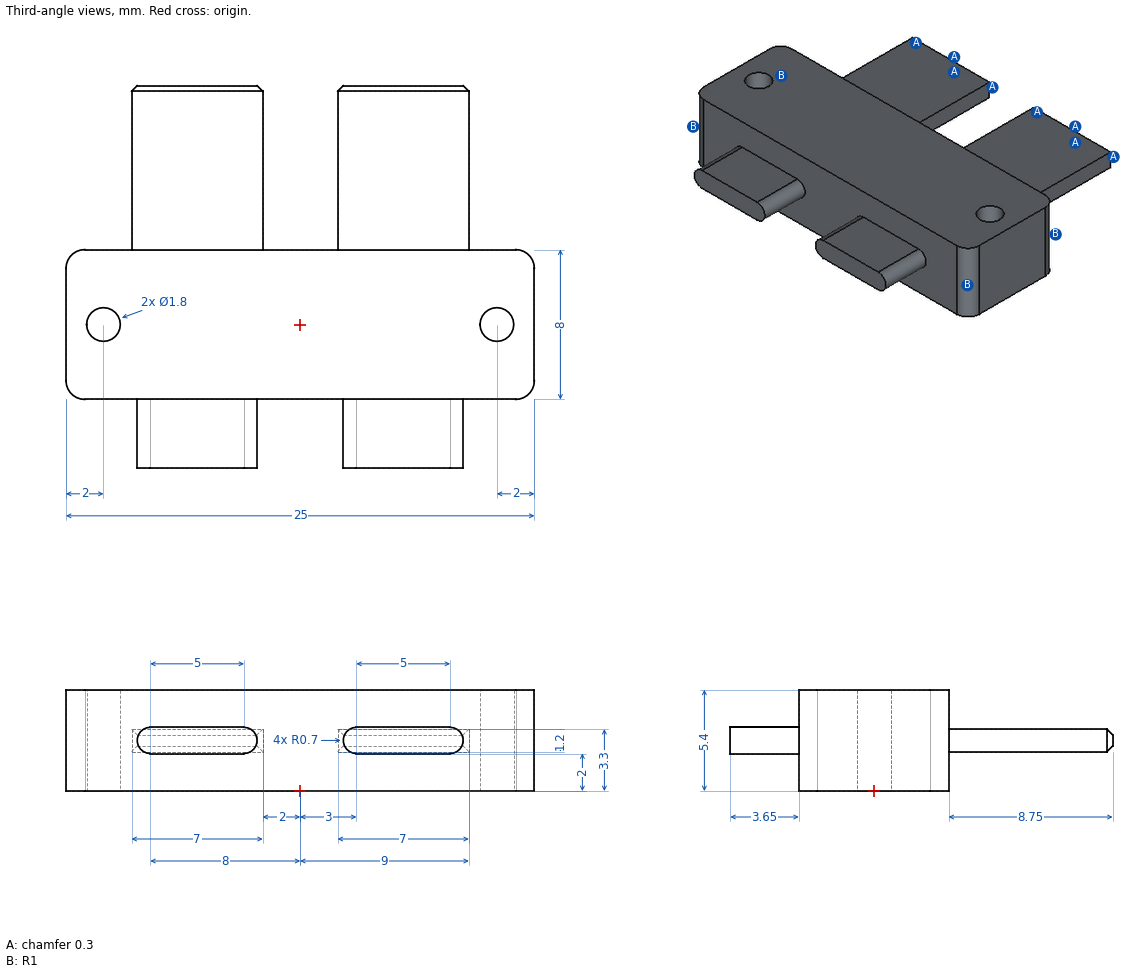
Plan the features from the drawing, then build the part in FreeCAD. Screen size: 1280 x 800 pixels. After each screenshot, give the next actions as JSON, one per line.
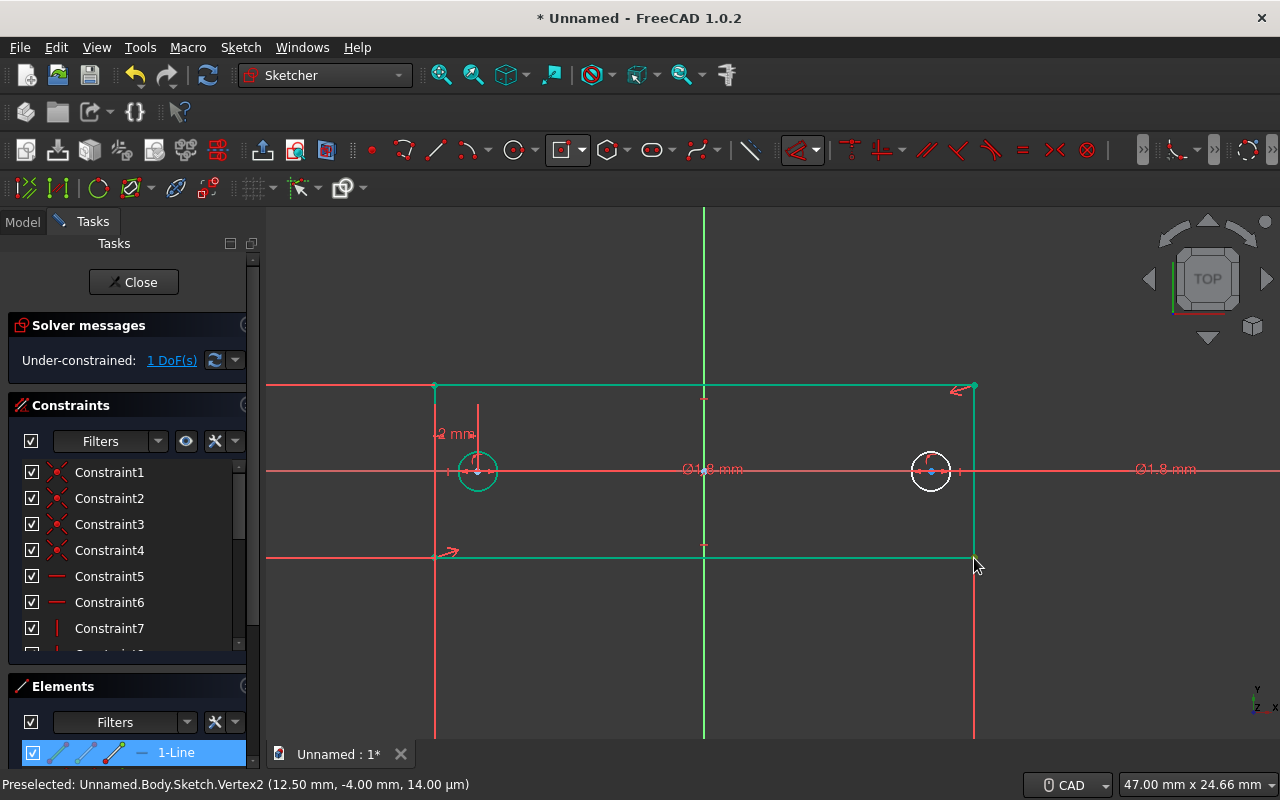
{"action": "left_click", "coordinate": [931, 471]}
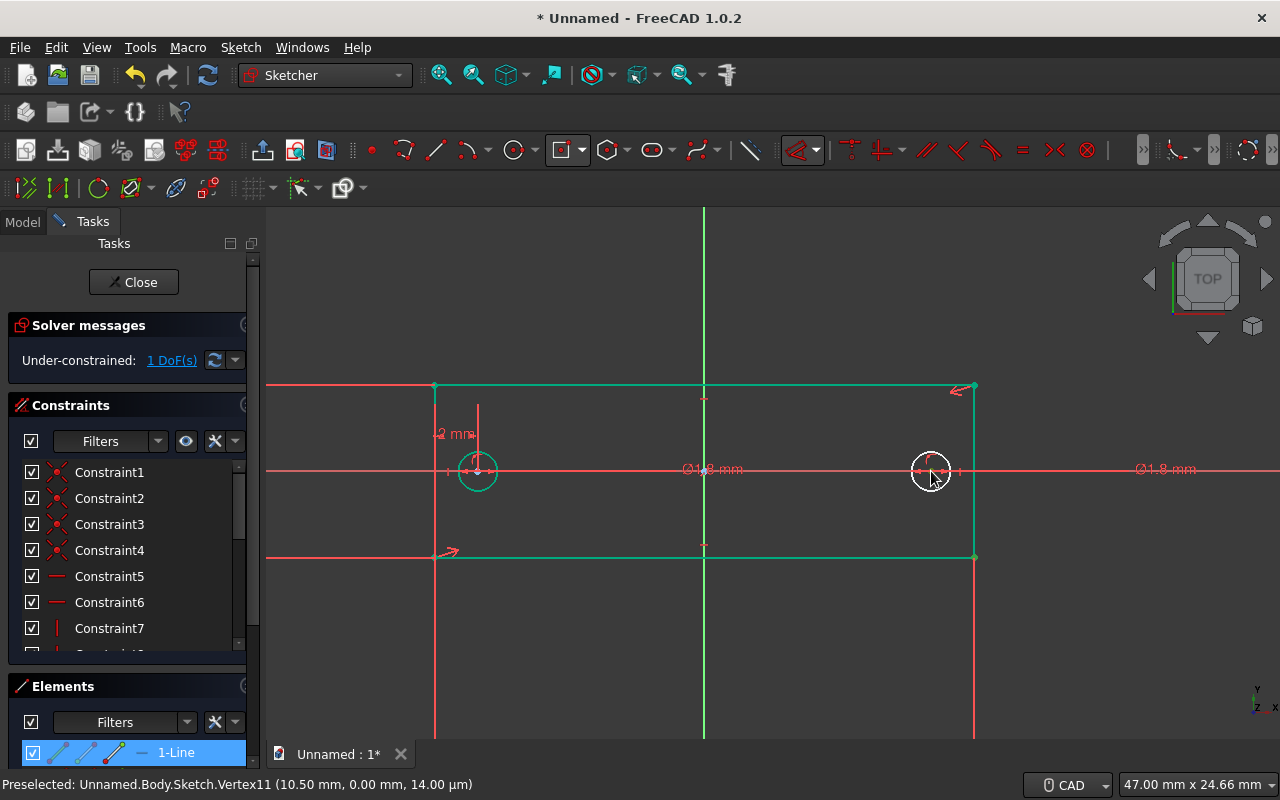
{"action": "key", "text": "l"}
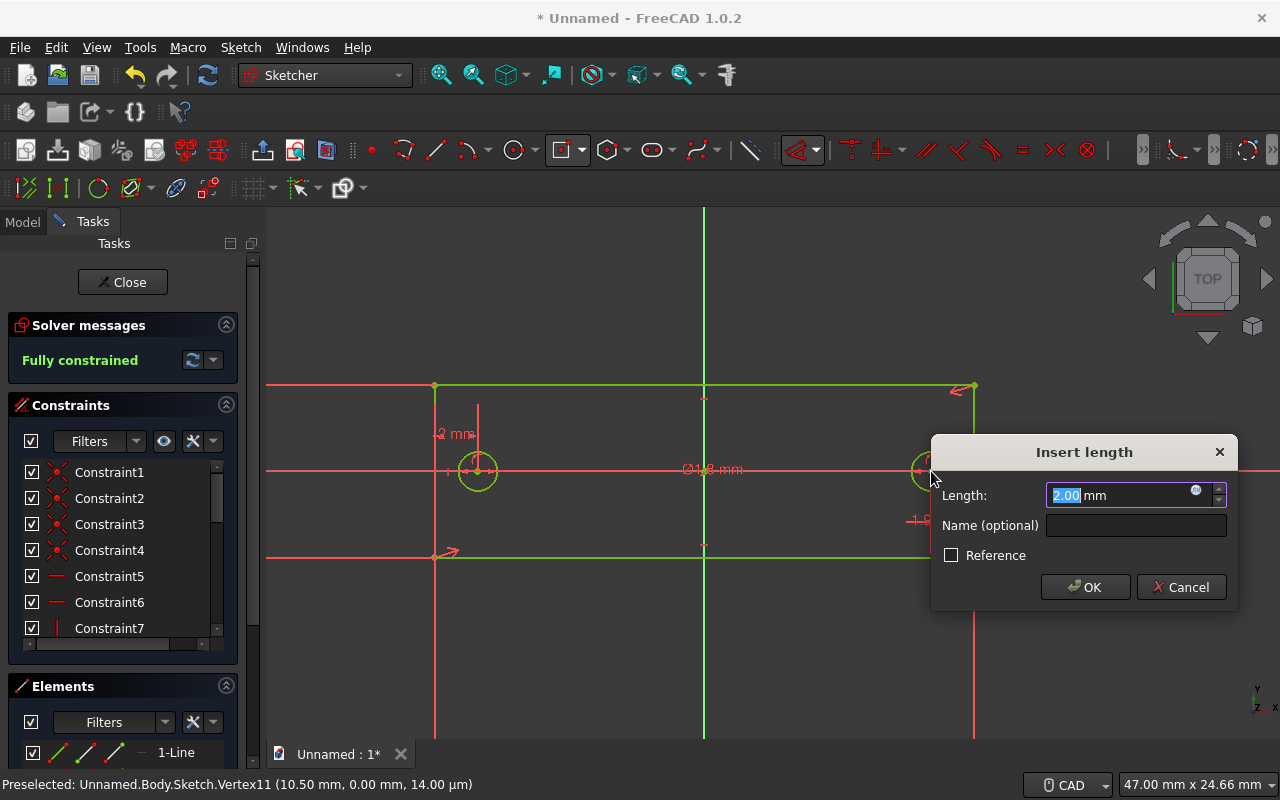
{"action": "type", "text": "2"}
{"action": "key", "text": "Return"}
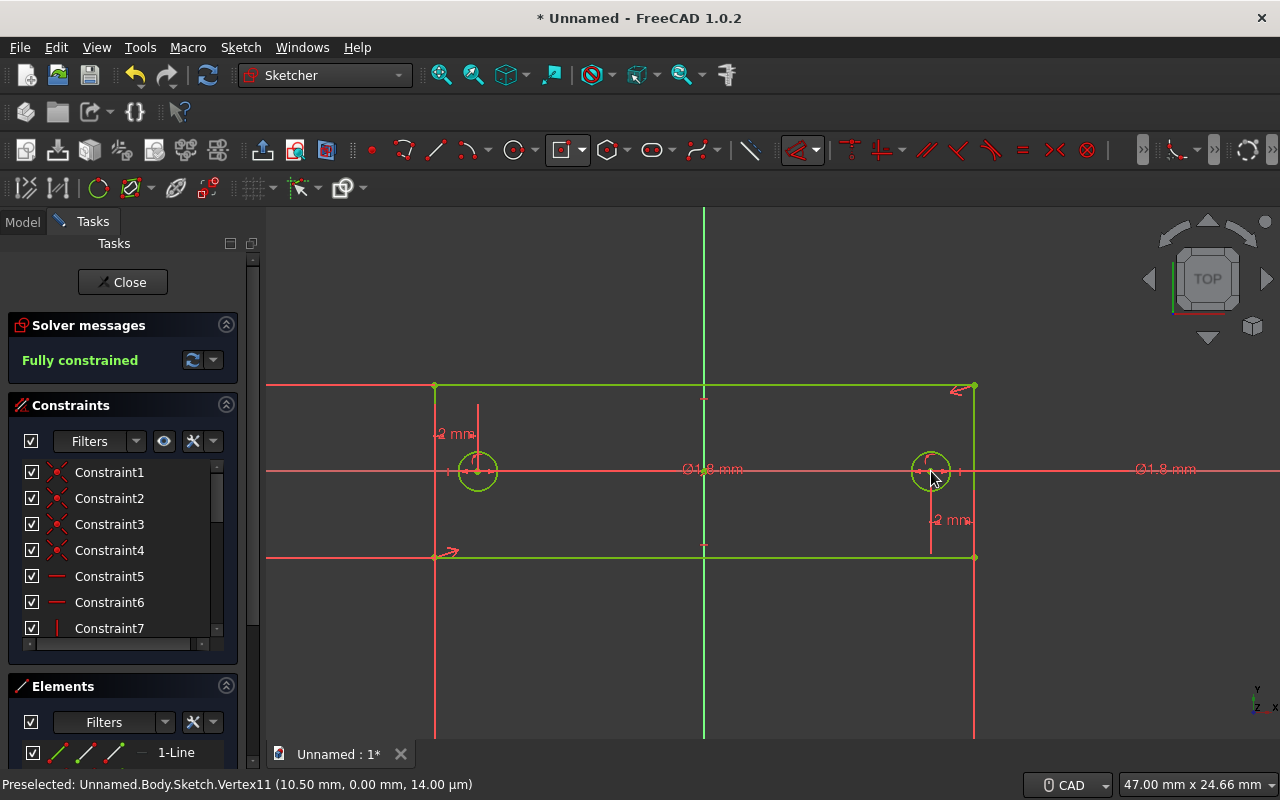
{"action": "left_click", "coordinate": [123, 282]}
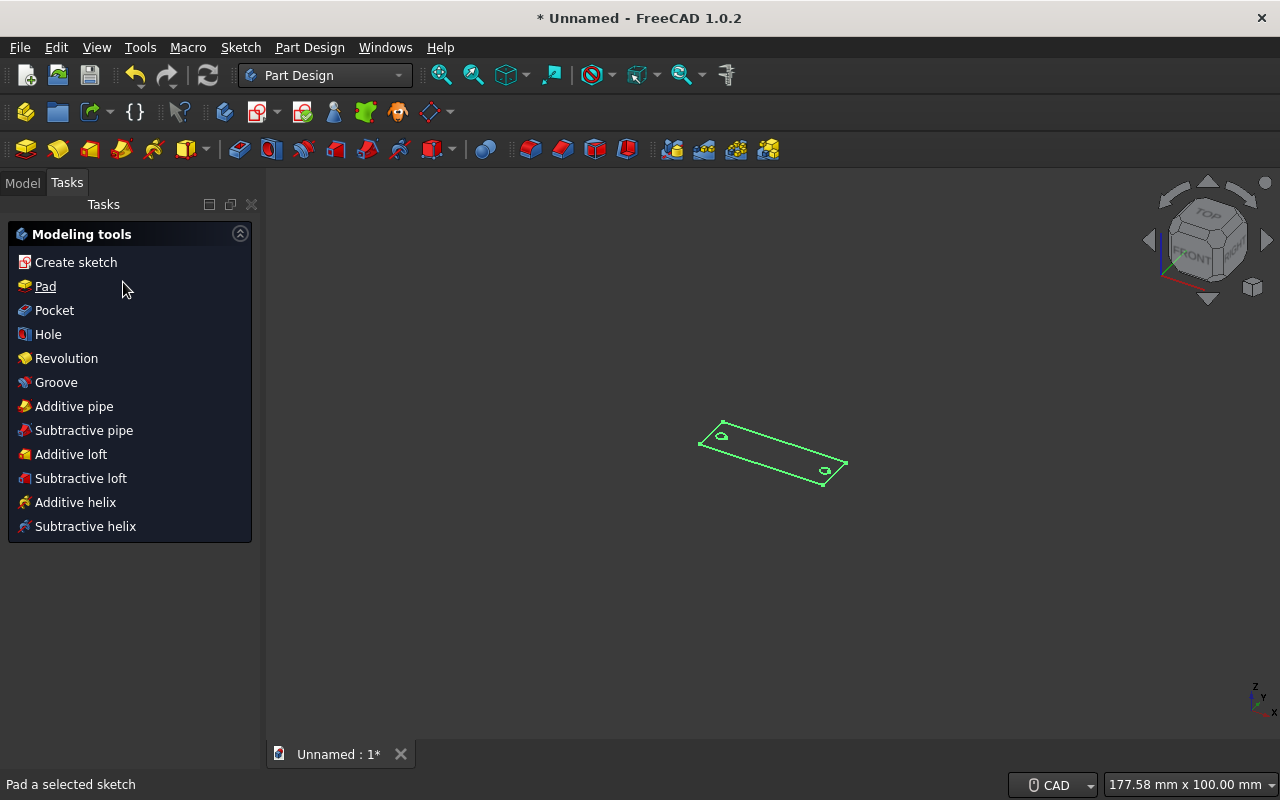
{"action": "left_click", "coordinate": [26, 150]}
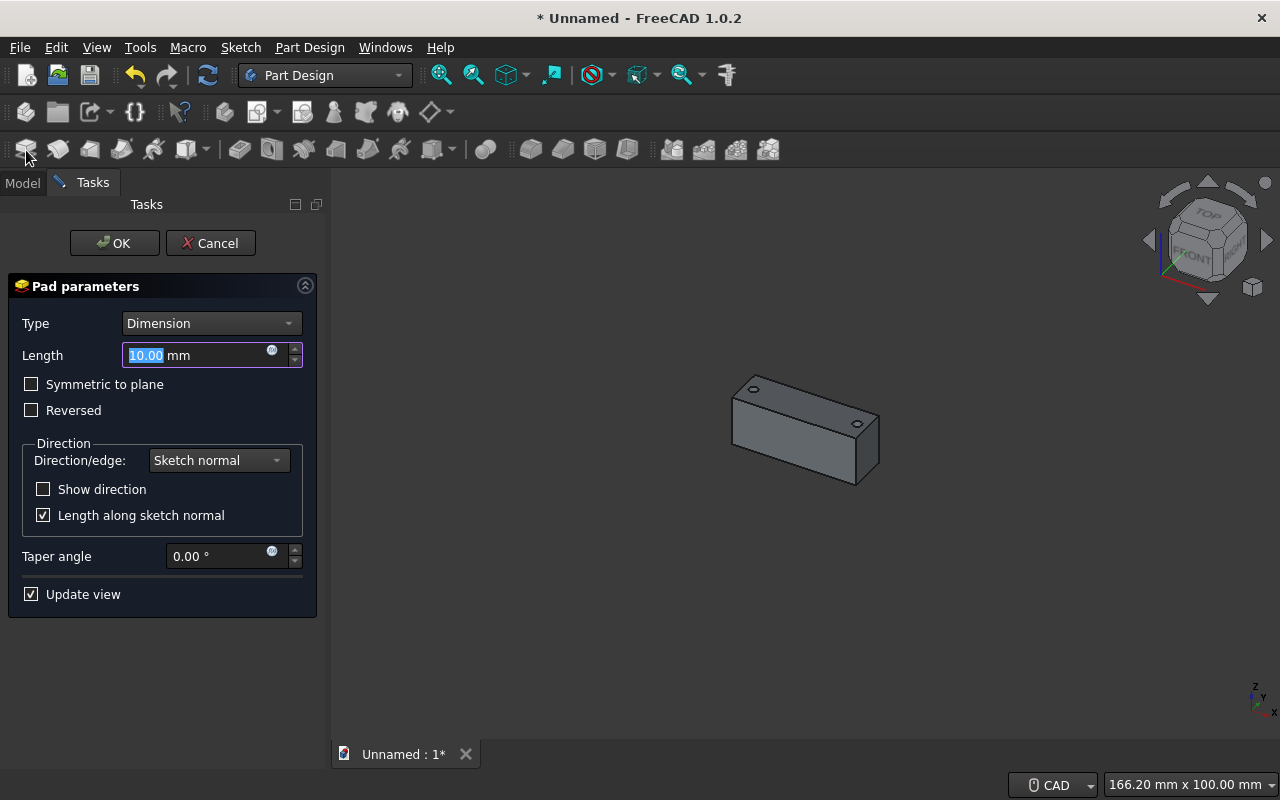
{"action": "type", "text": "5.4"}
{"action": "key", "text": "Tab"}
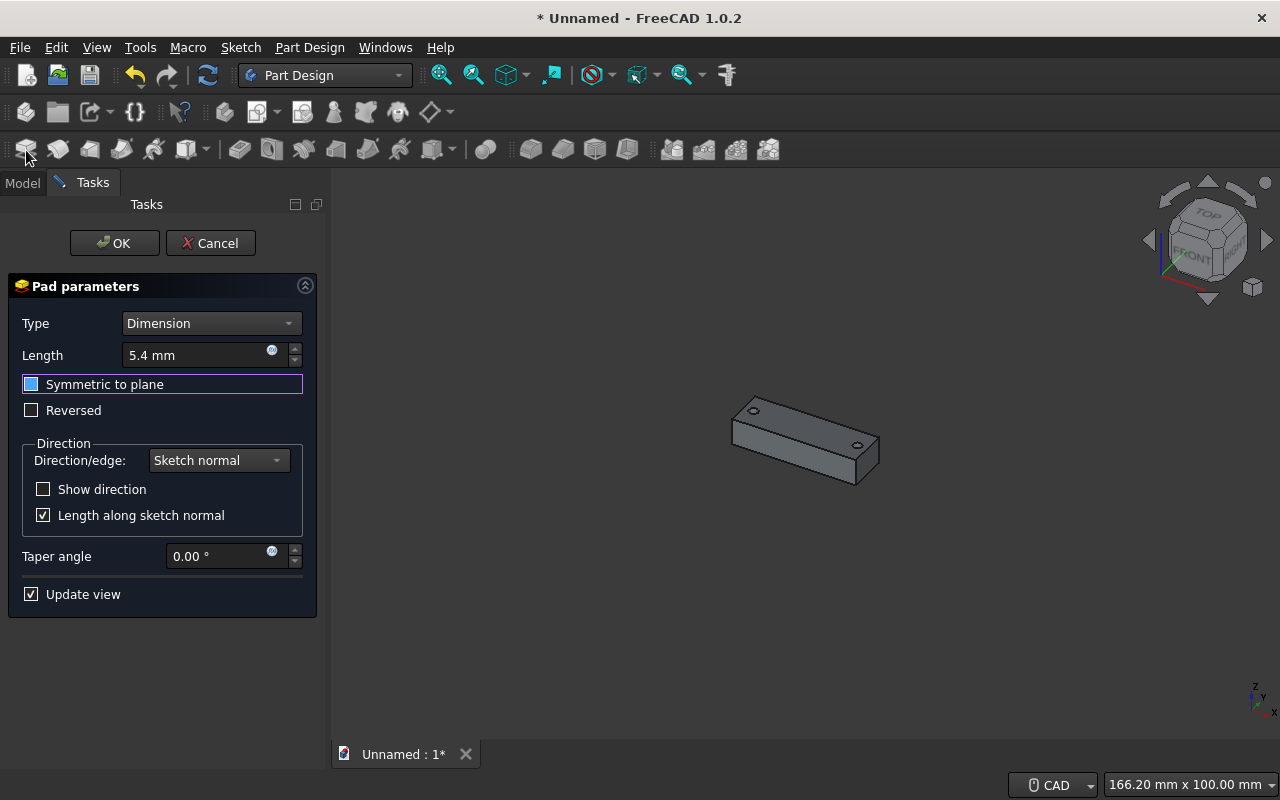
{"action": "left_click", "coordinate": [115, 243]}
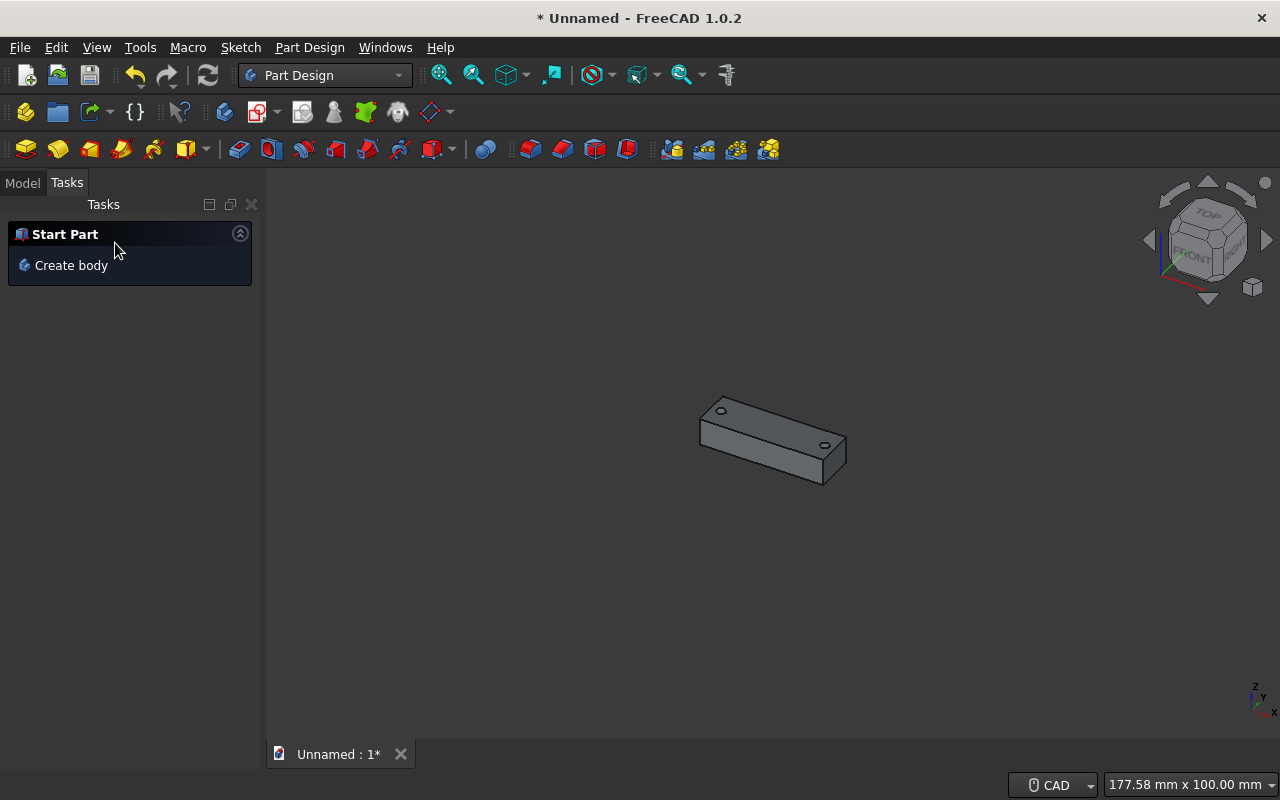
{"action": "left_click", "coordinate": [442, 76]}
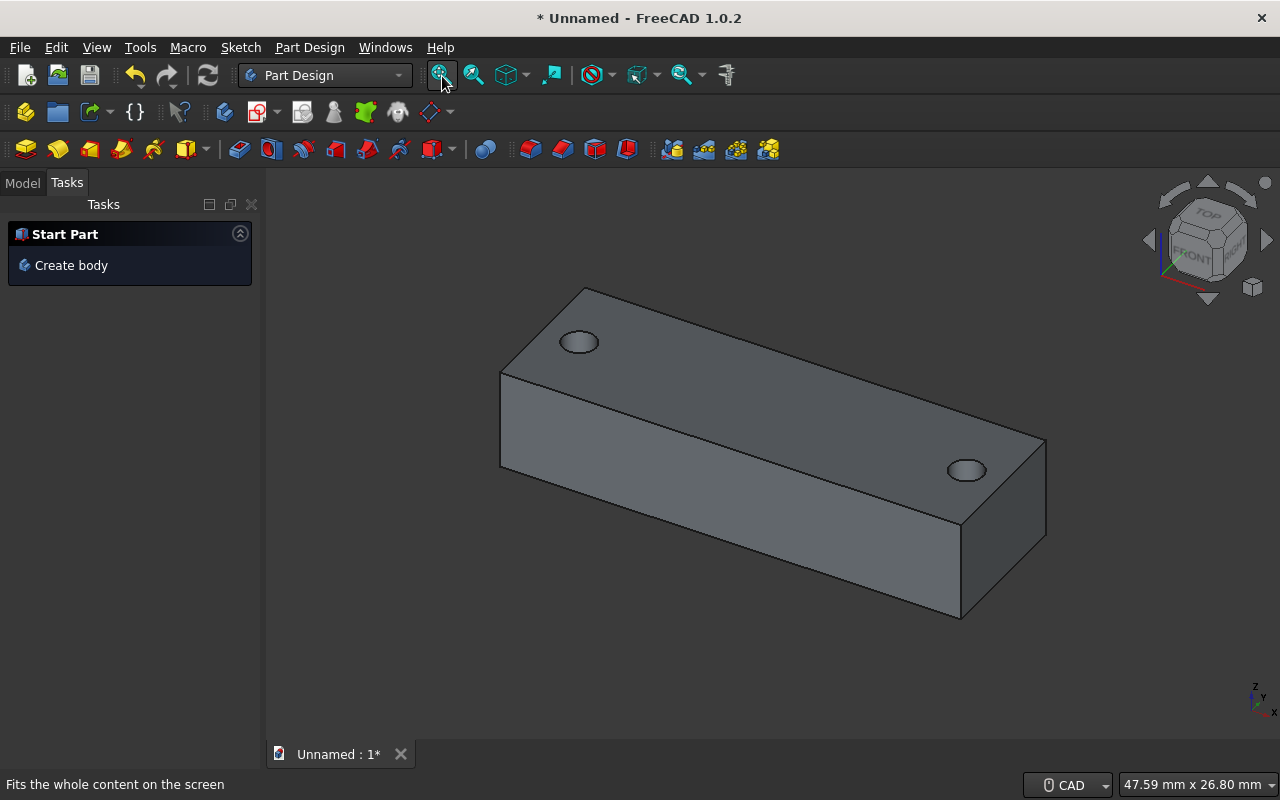
{"action": "left_click", "coordinate": [862, 538]}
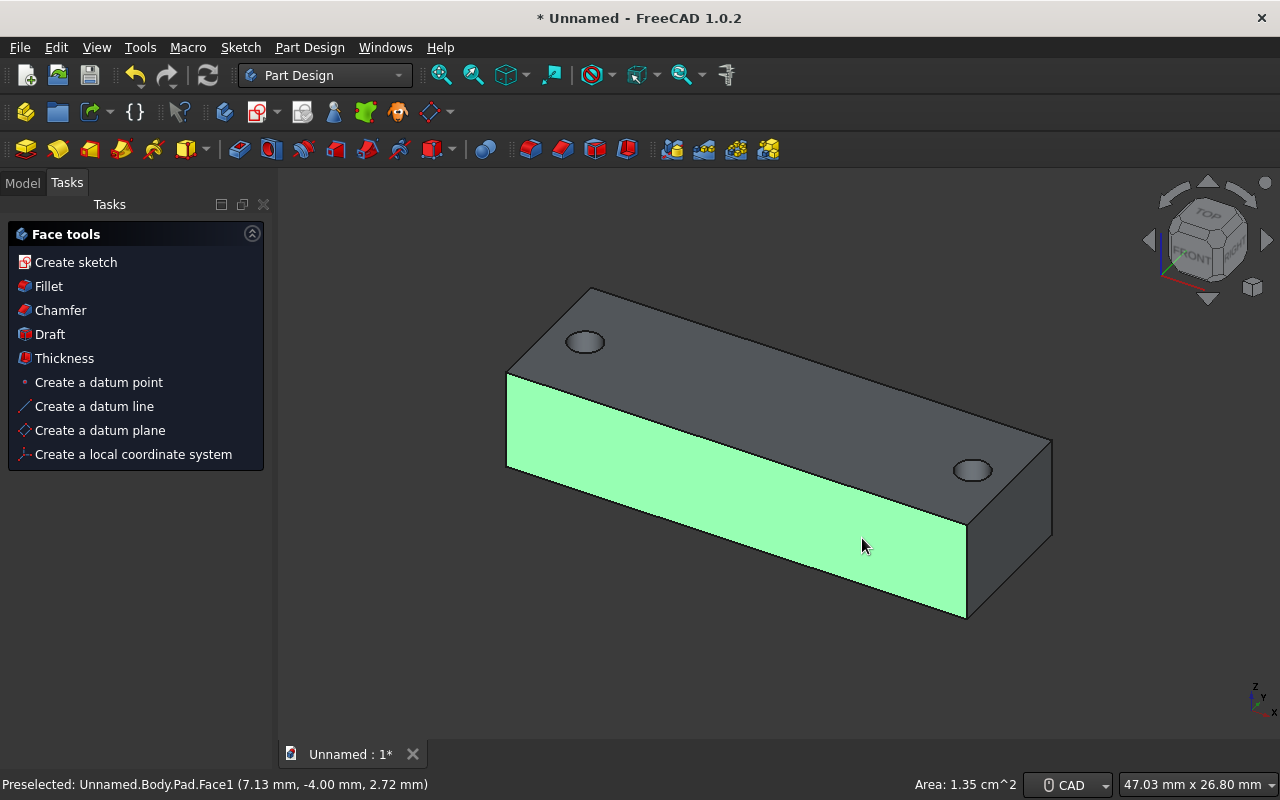
{"action": "left_click", "coordinate": [258, 112]}